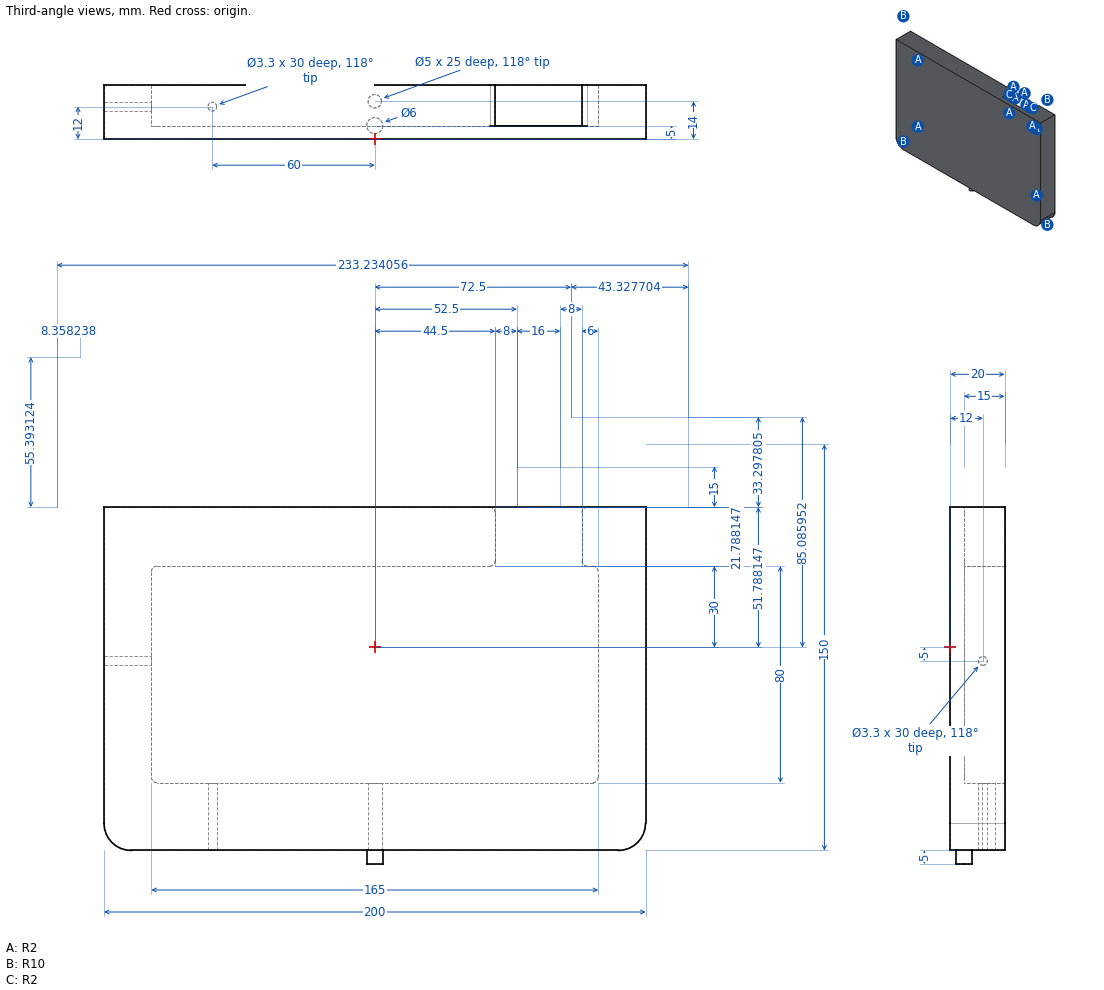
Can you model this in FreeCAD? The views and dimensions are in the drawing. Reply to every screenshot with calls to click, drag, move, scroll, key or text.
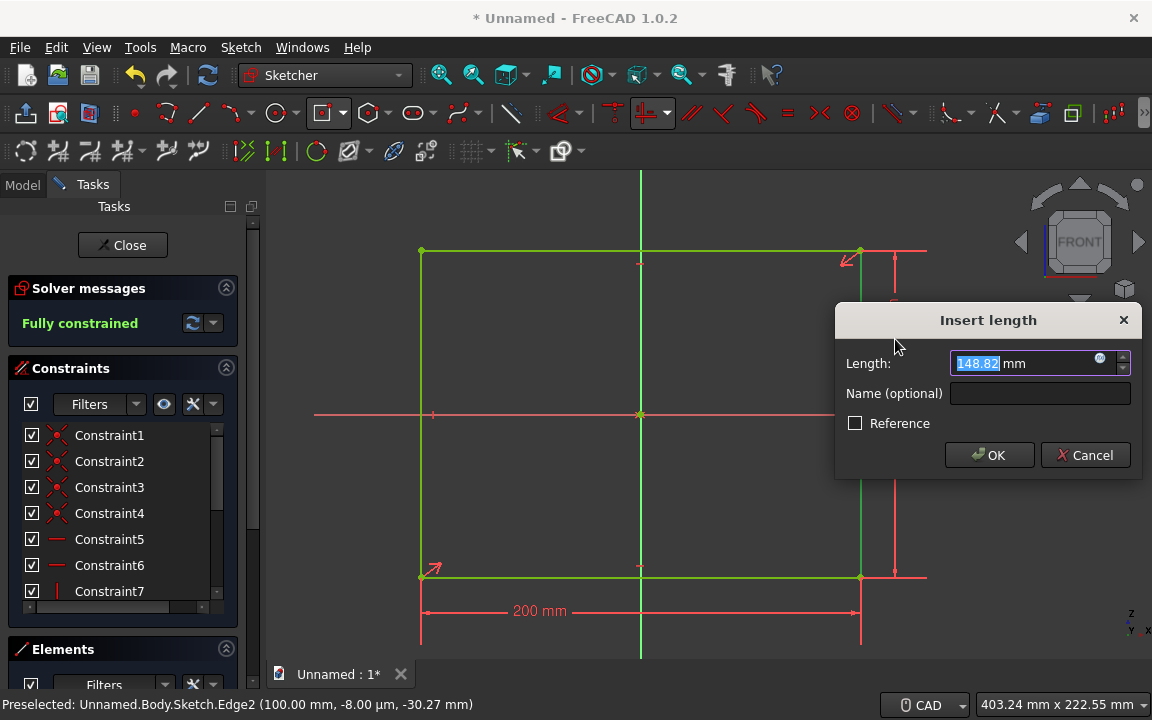
text(150)
key(Return)
key(Escape)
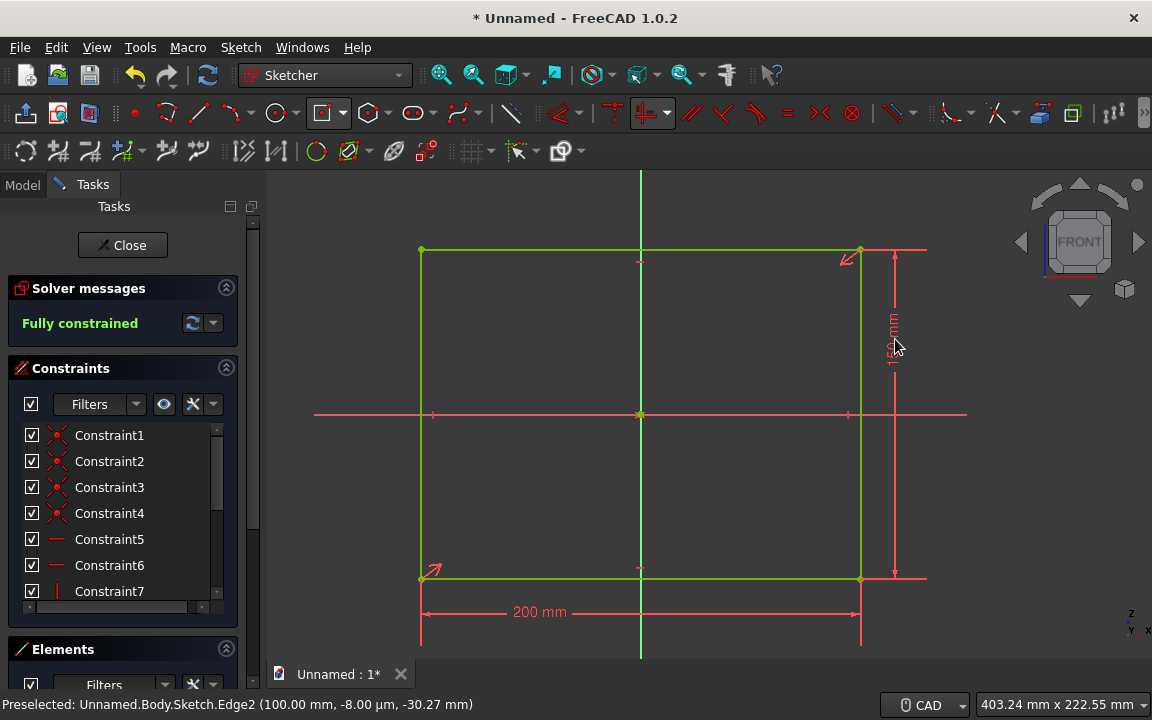
click(123, 245)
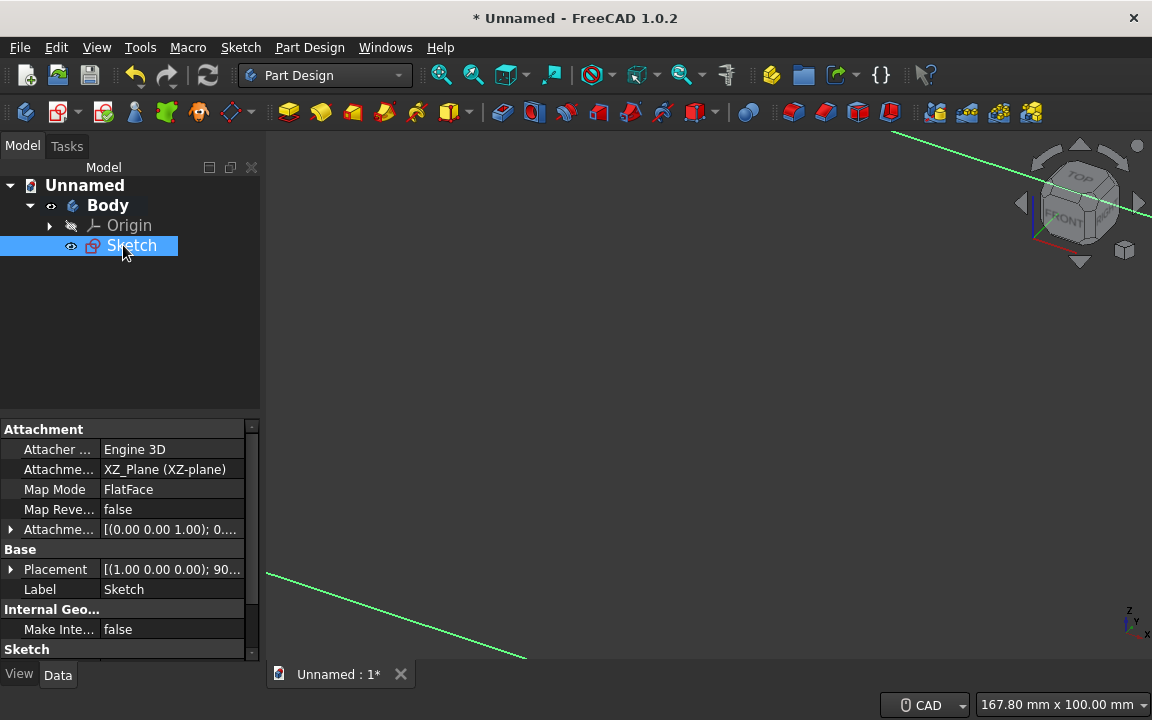
click(290, 112)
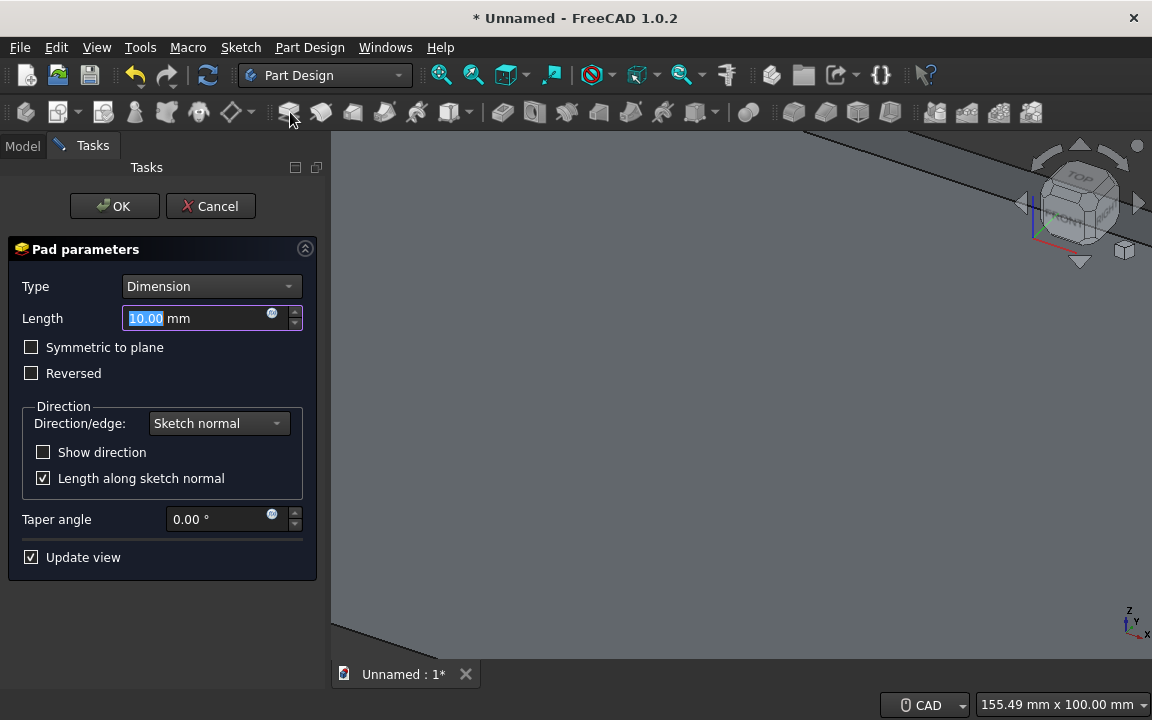
text(20)
key(Tab)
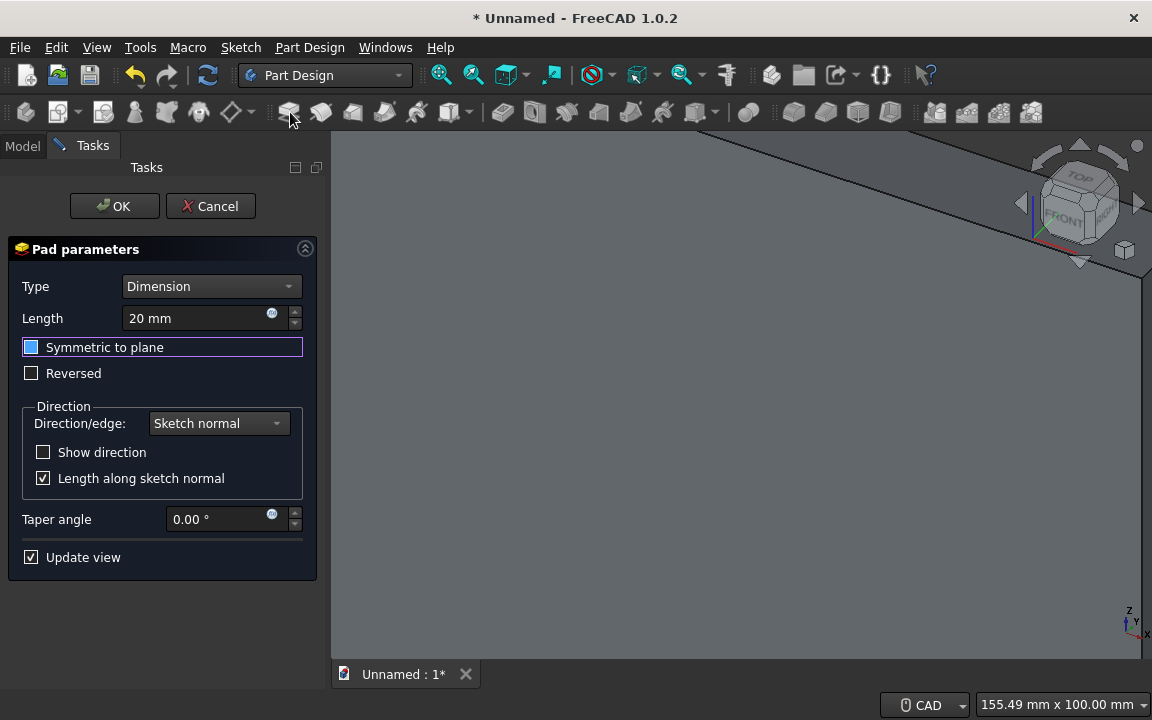
click(30, 373)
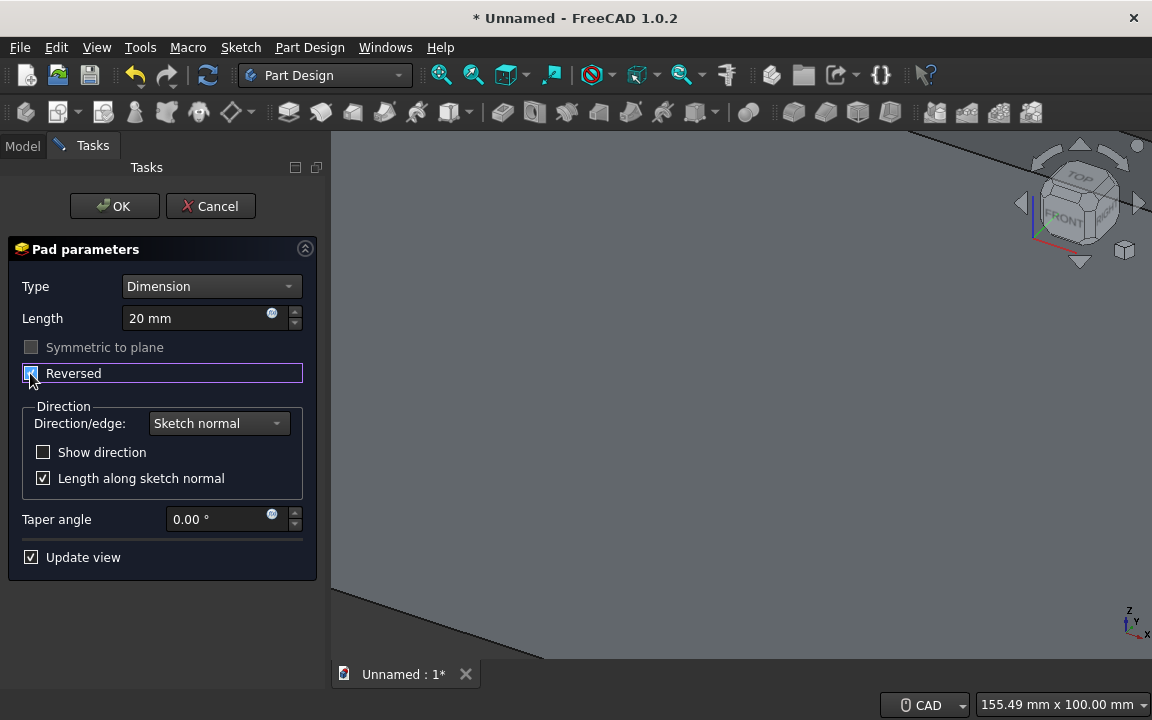
click(115, 206)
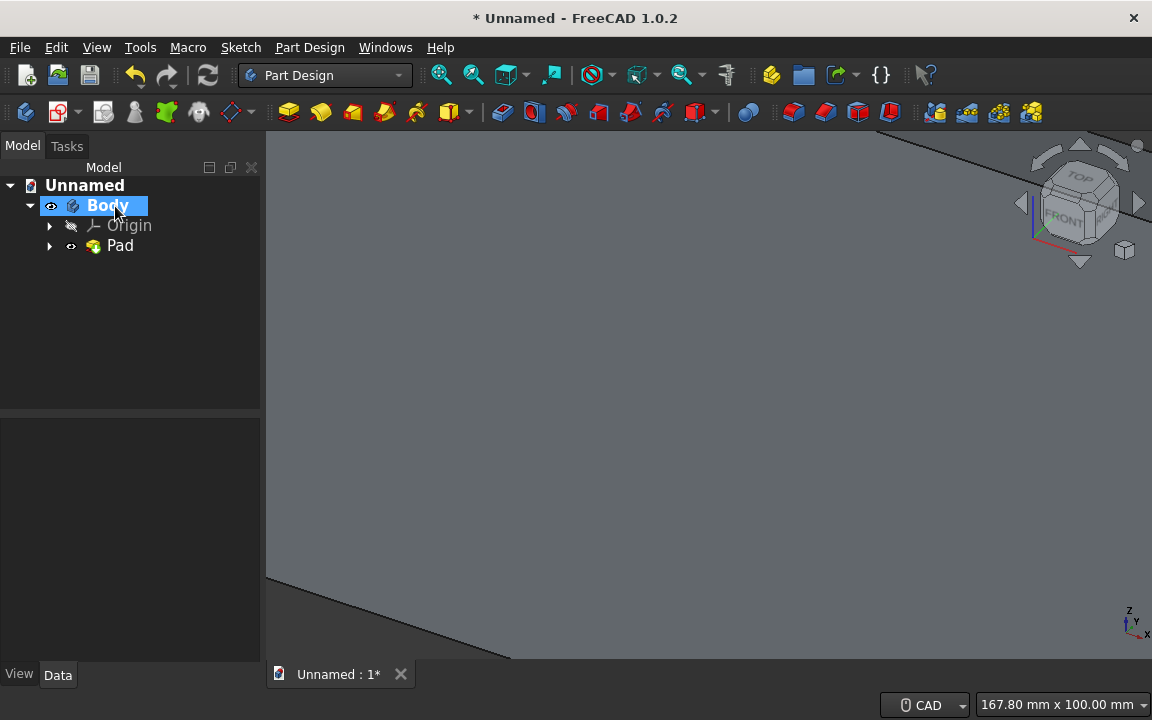
key(v)
key(f)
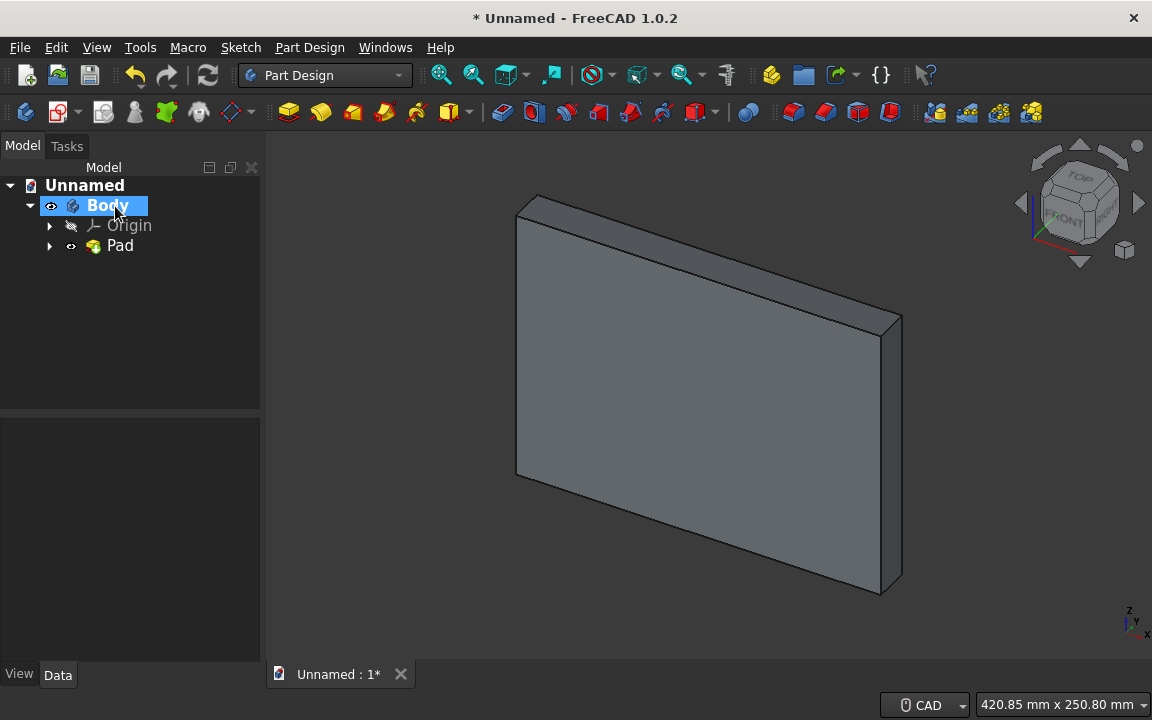
key(5)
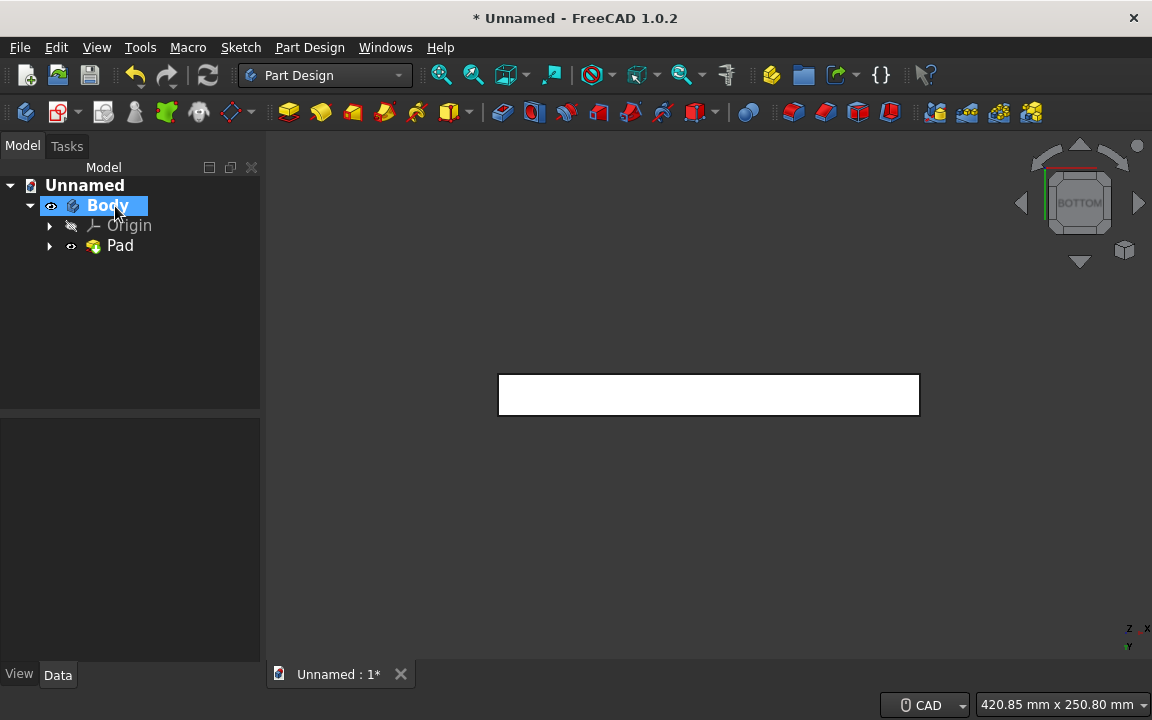
click(889, 394)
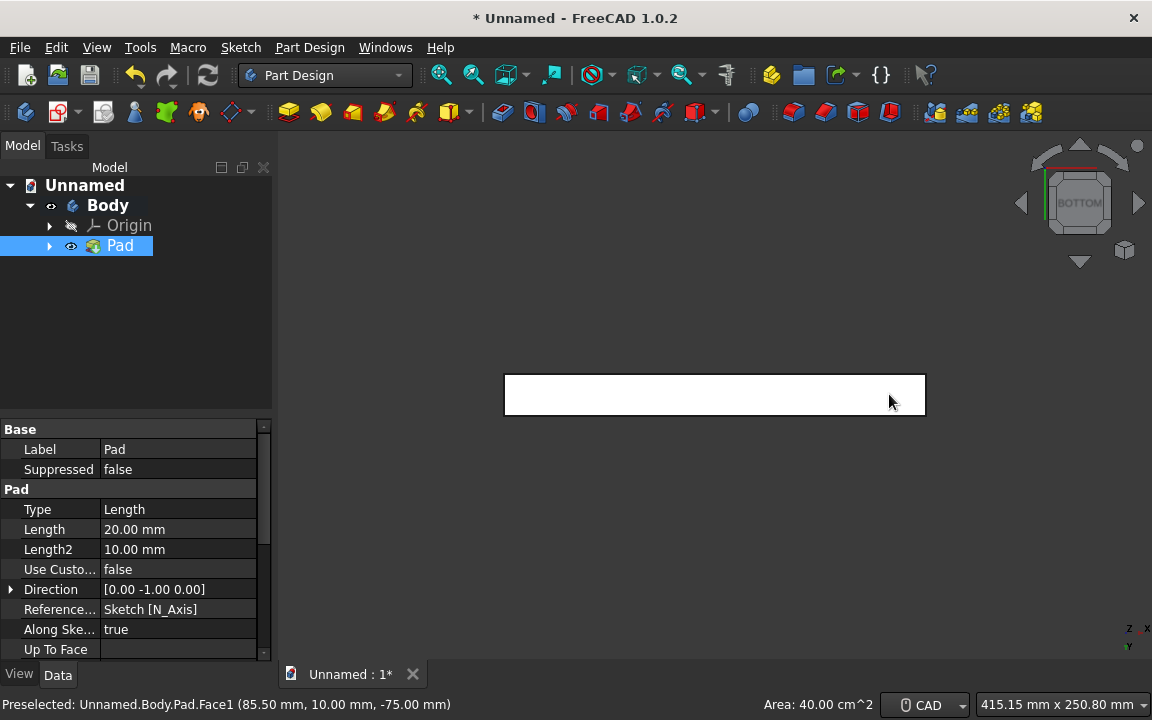
click(58, 112)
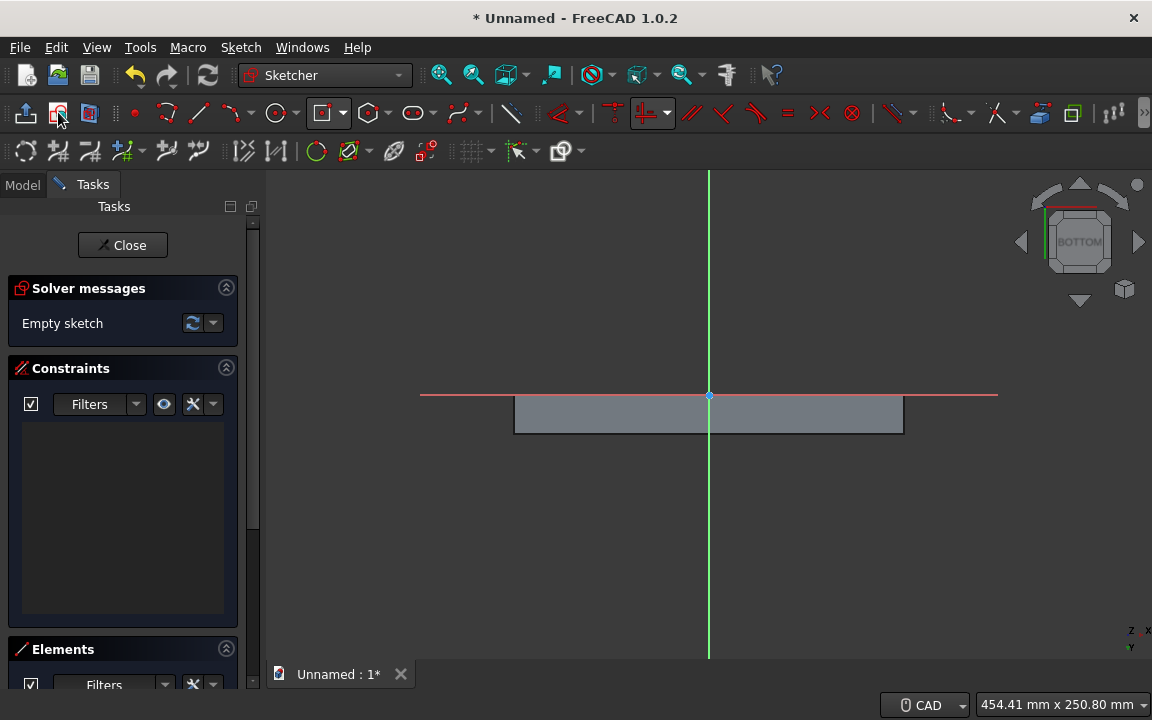
scroll(713, 402, up, 15)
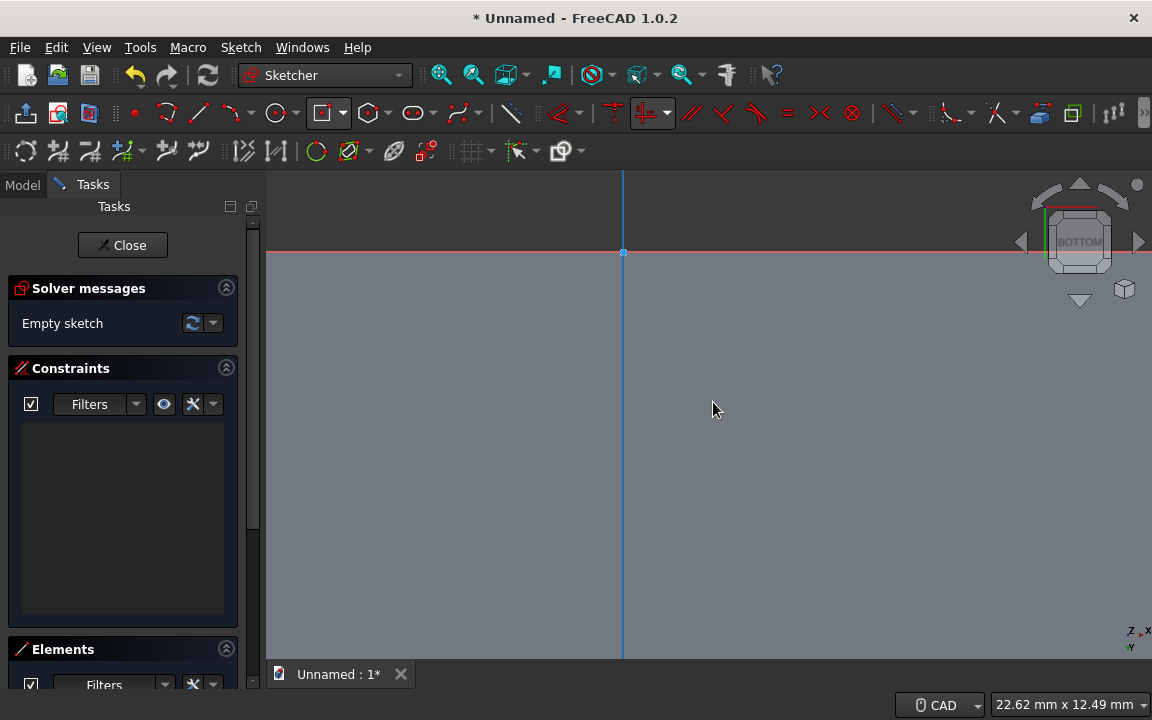
click(276, 114)